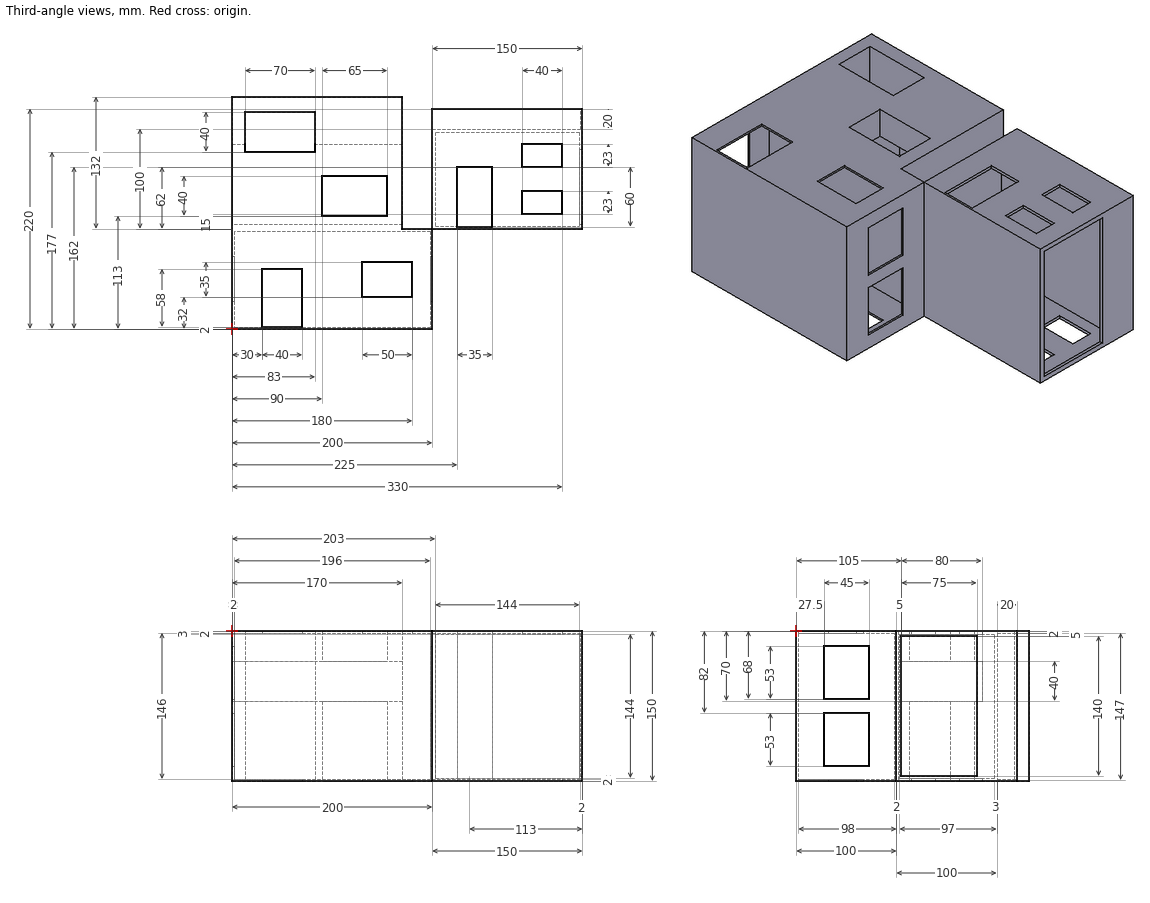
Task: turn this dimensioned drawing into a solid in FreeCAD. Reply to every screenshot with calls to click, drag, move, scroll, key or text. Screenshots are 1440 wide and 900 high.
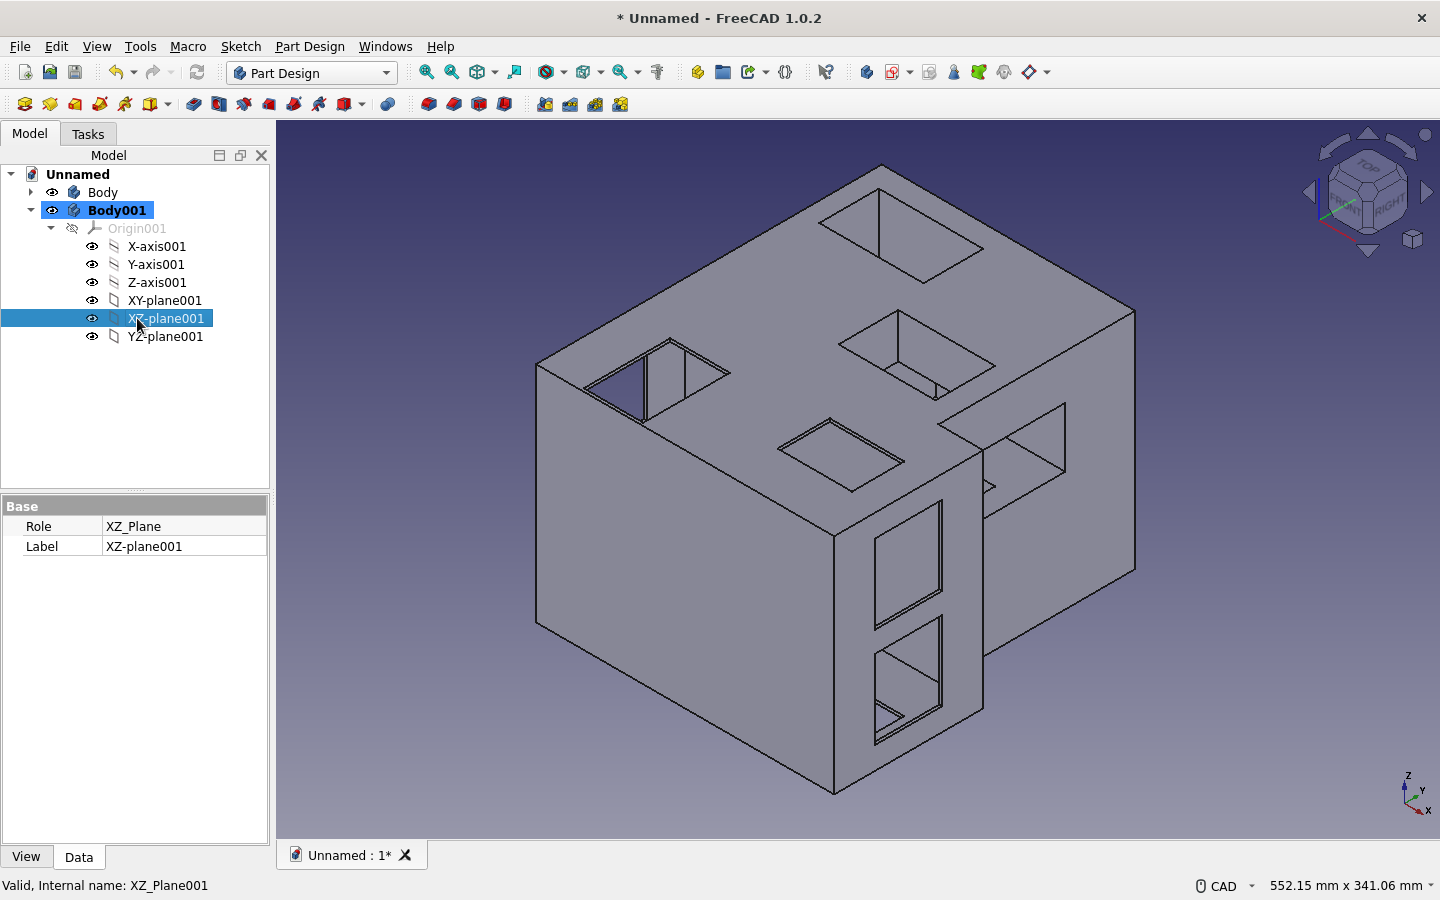
click(1028, 72)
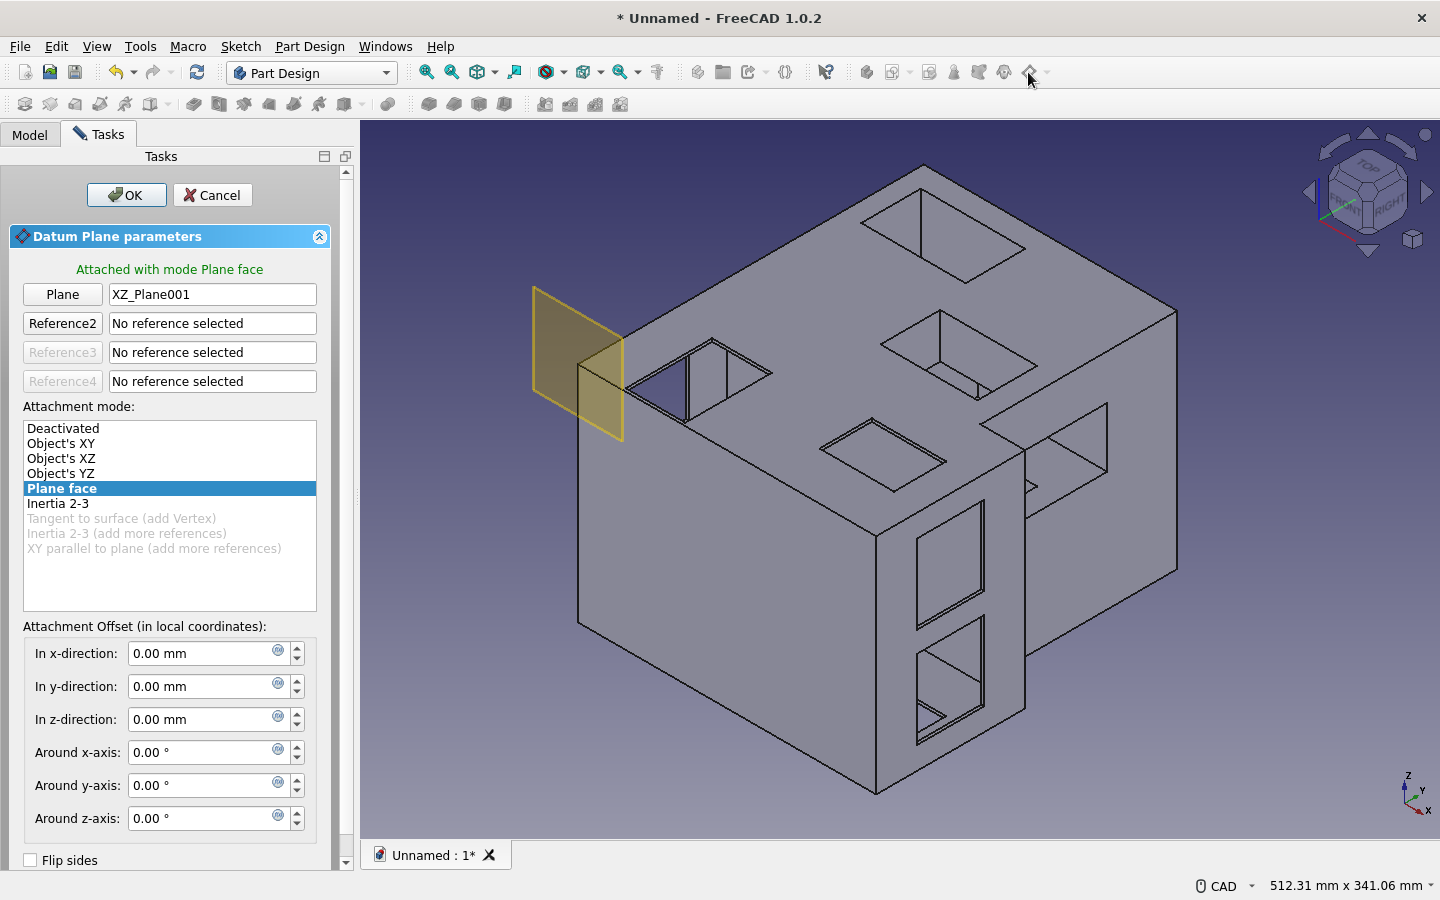
triple_click(210, 720)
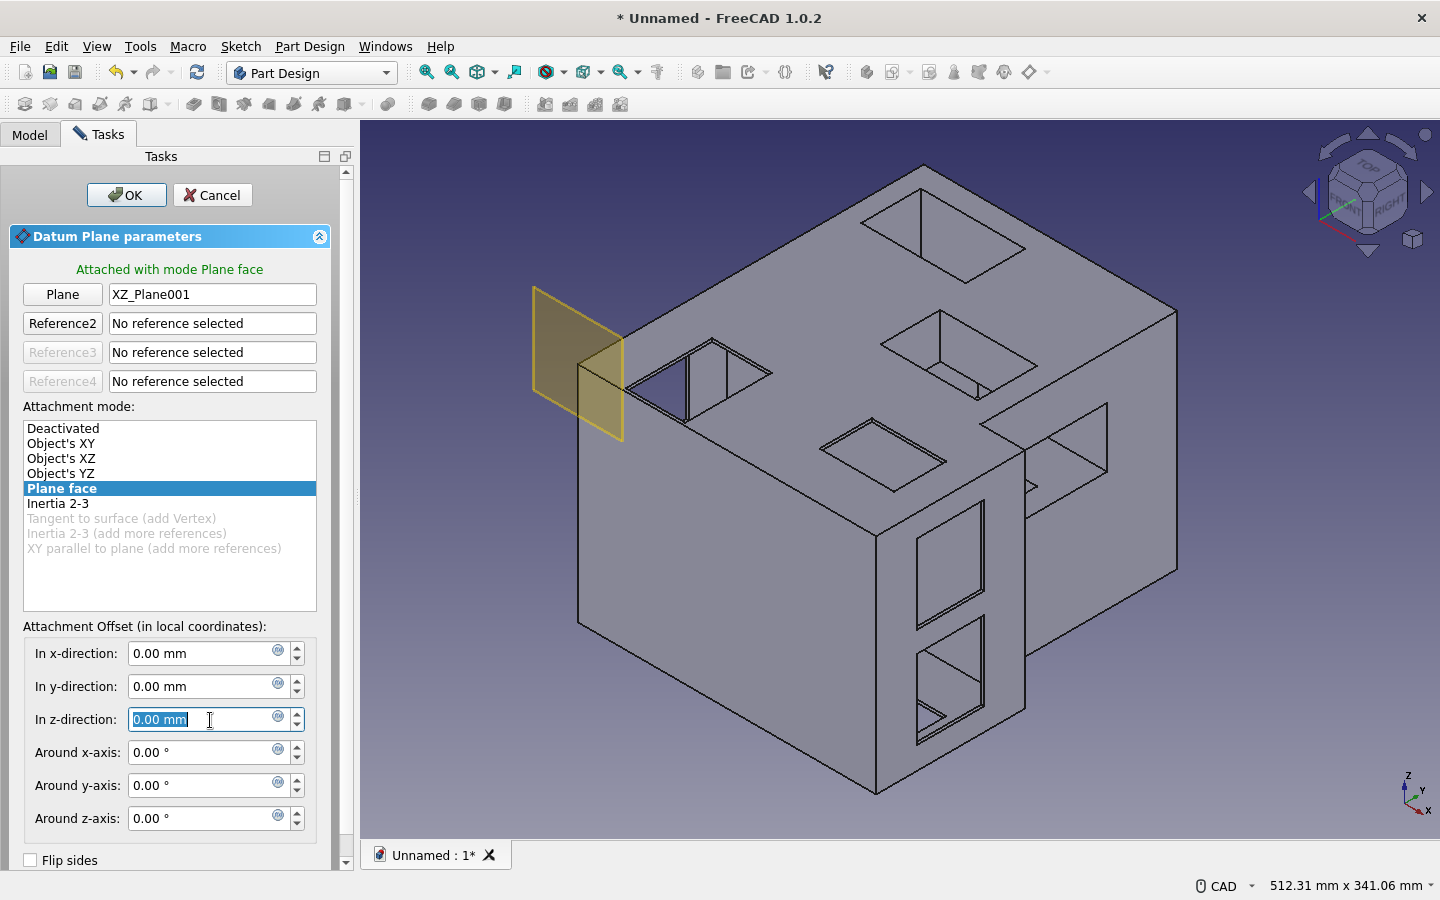
text(-100)
key(Tab)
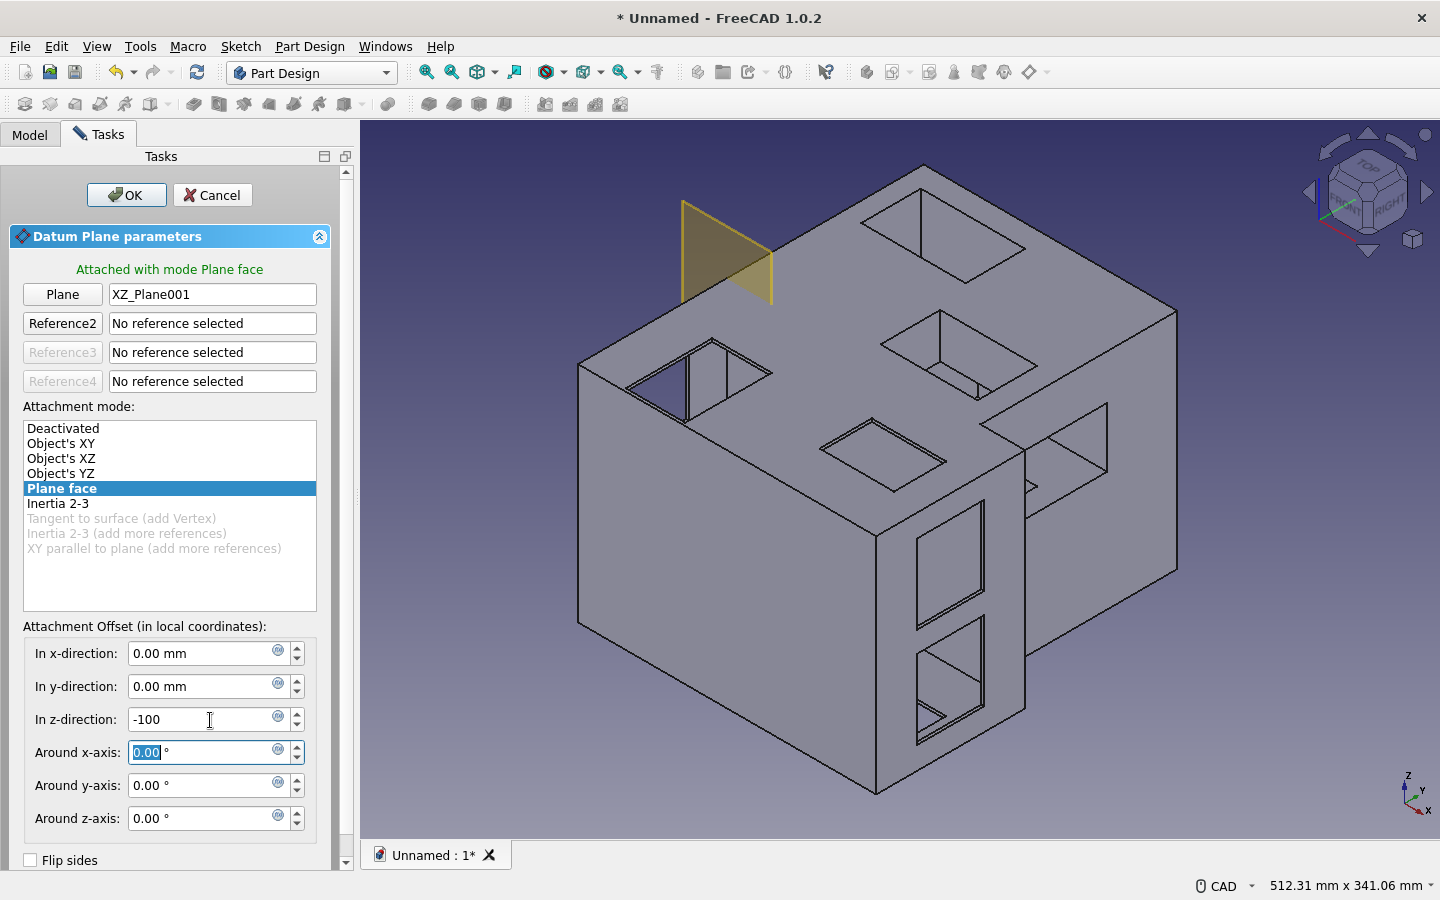
click(127, 195)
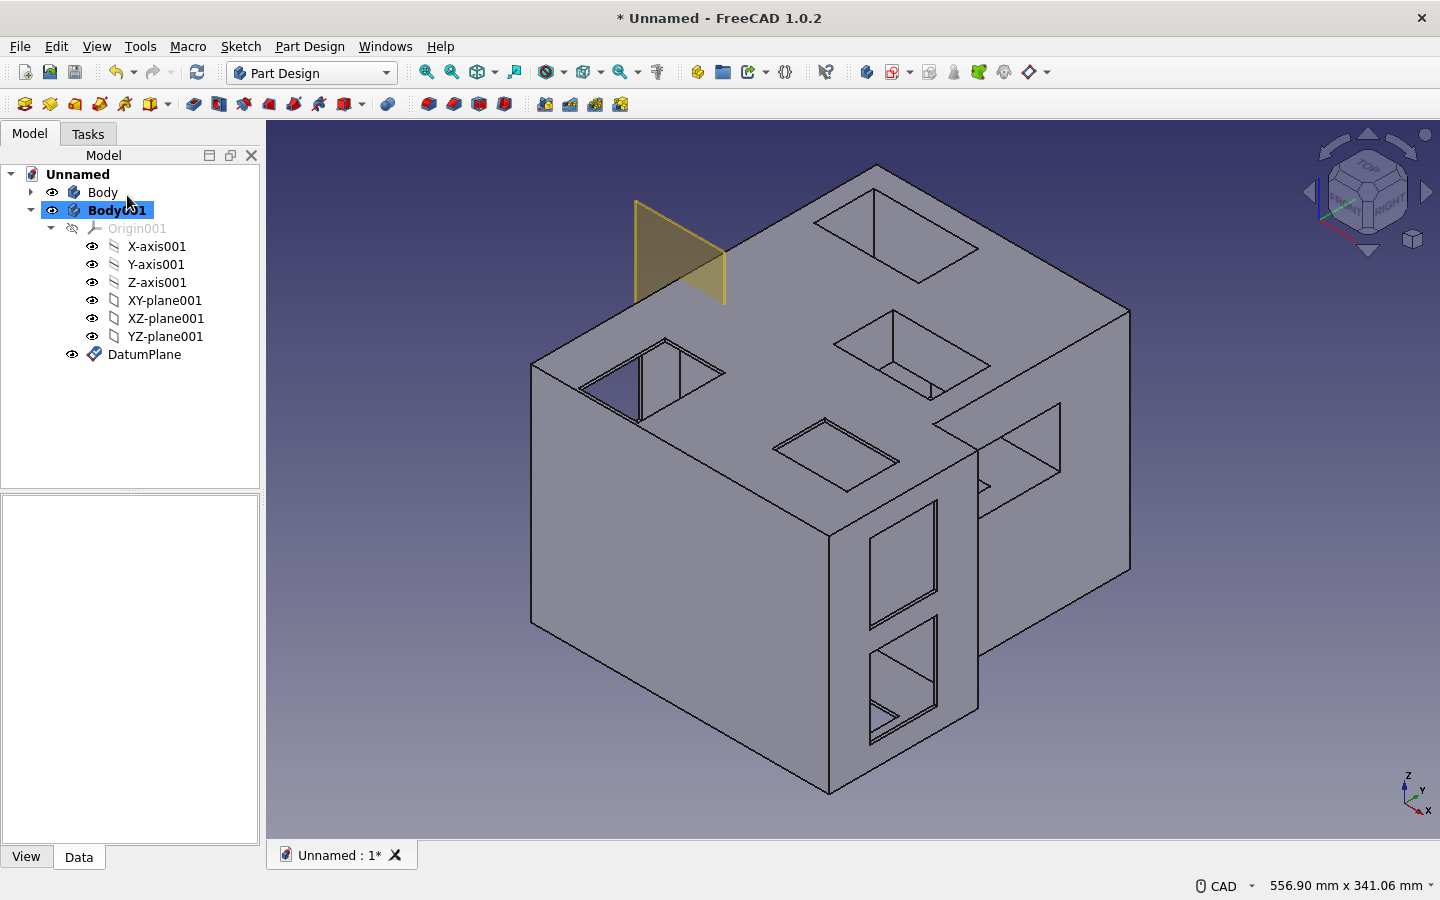
click(117, 354)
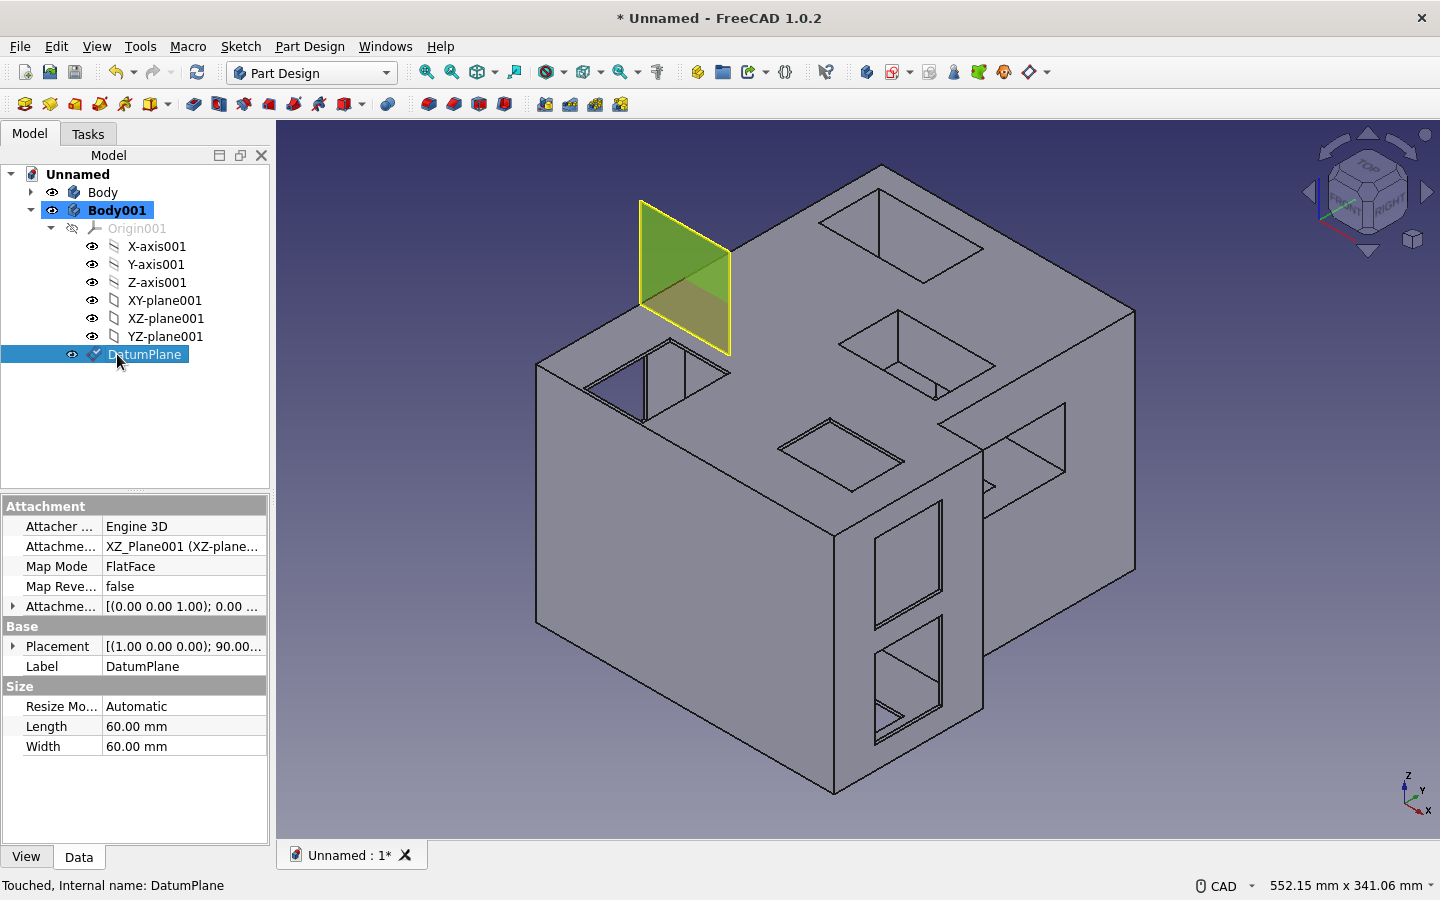
click(892, 72)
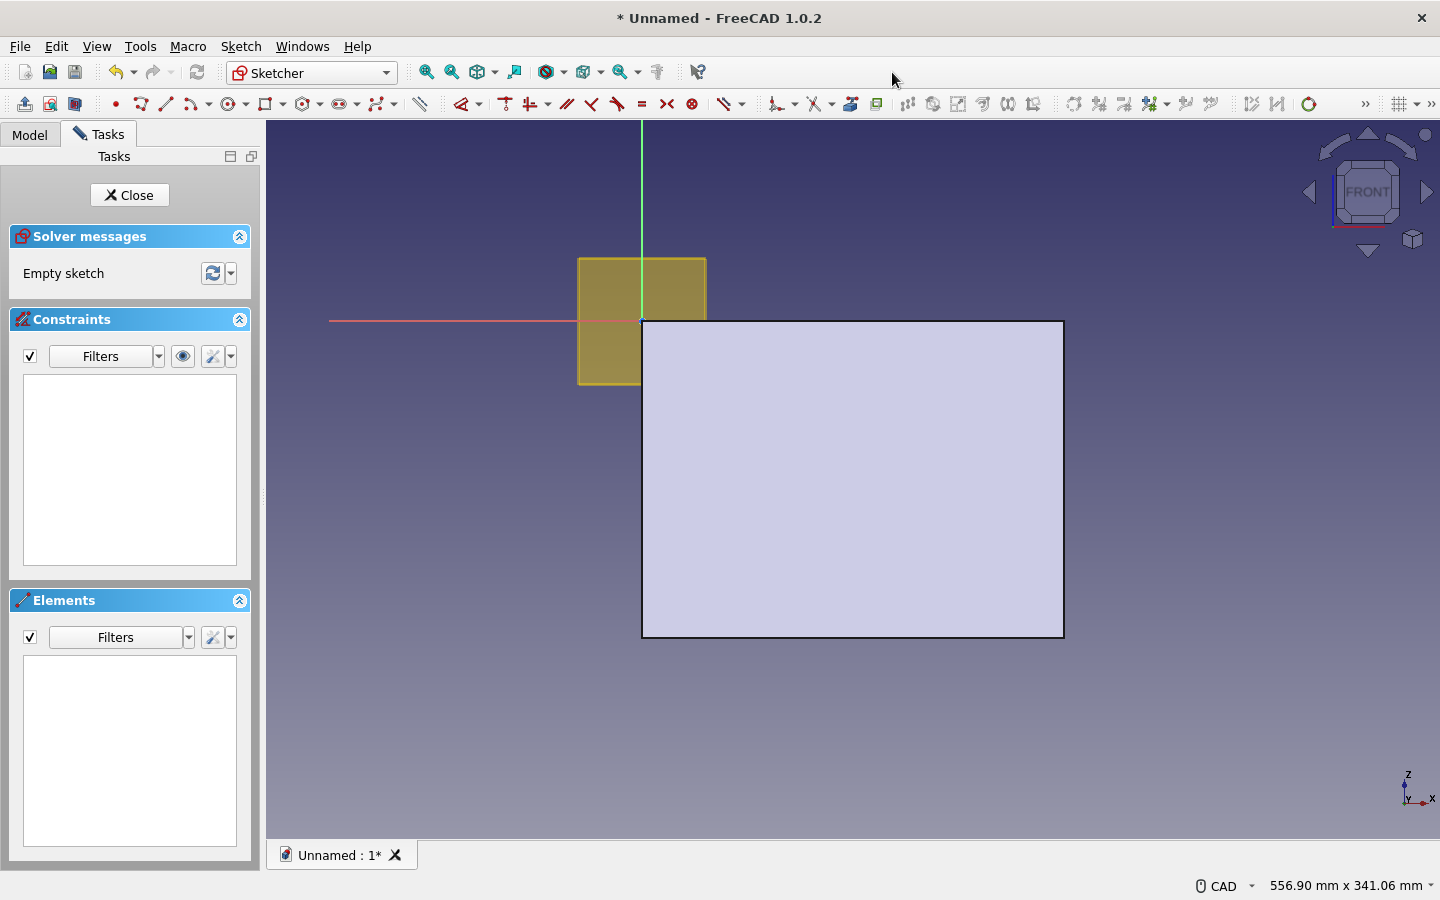
scroll(294, 479, down, 1)